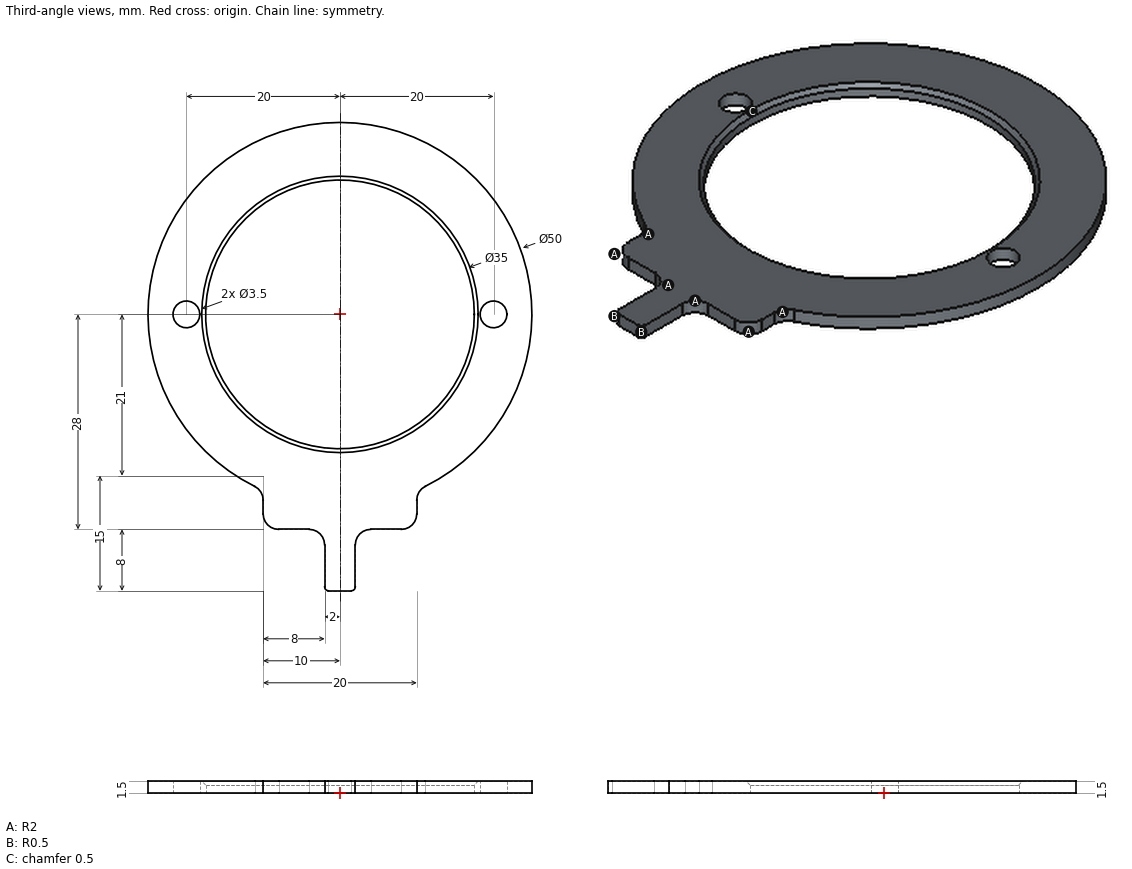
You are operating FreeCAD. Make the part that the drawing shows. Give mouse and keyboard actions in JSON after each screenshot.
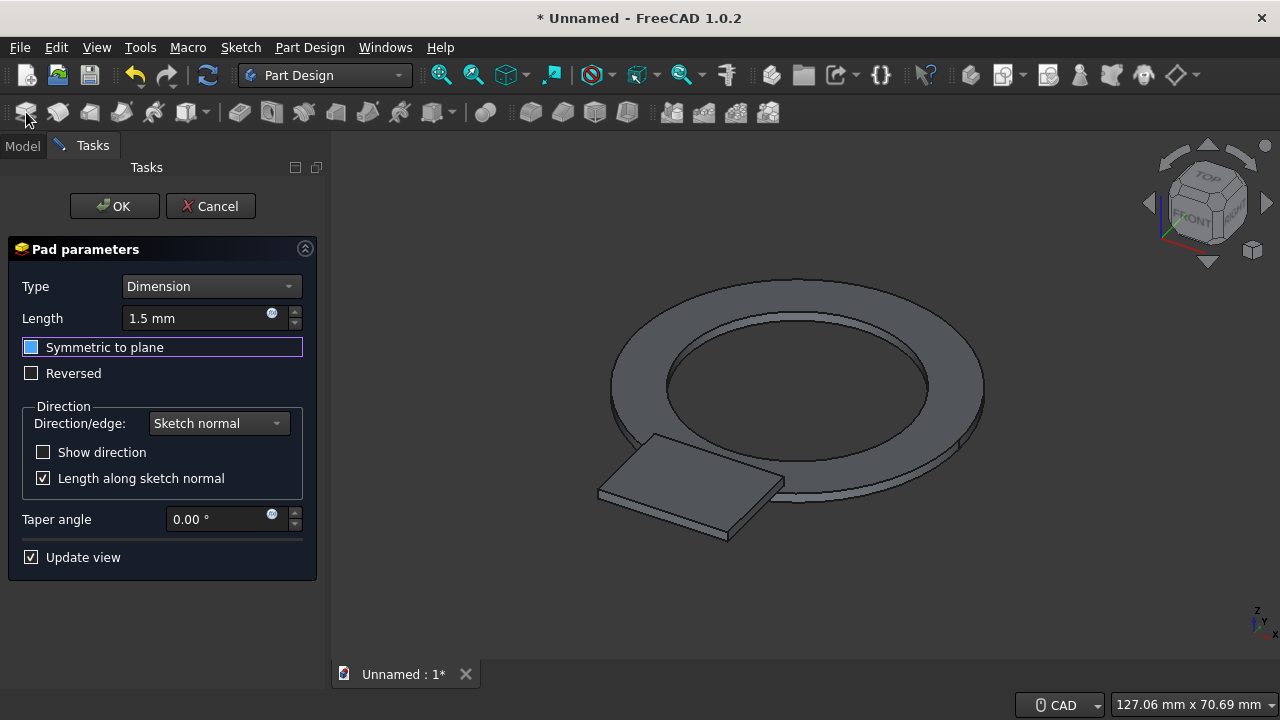
{"action": "left_click", "coordinate": [30, 373]}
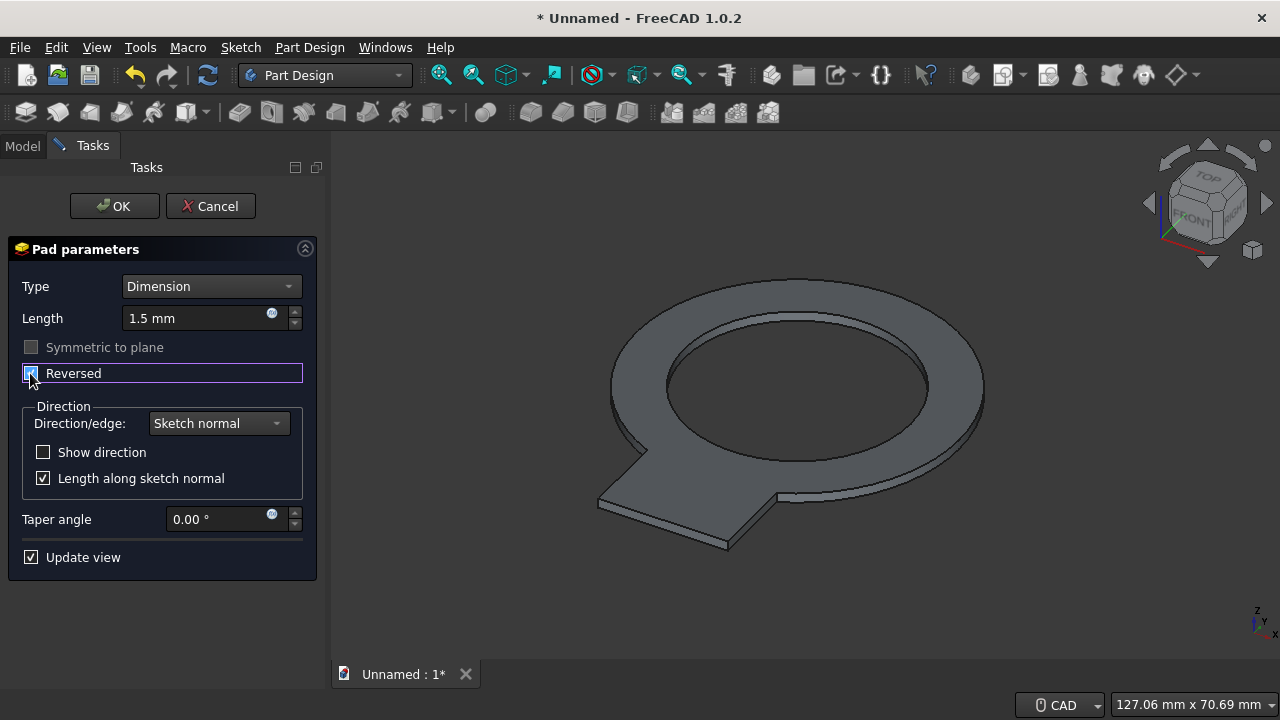
{"action": "left_click", "coordinate": [115, 206]}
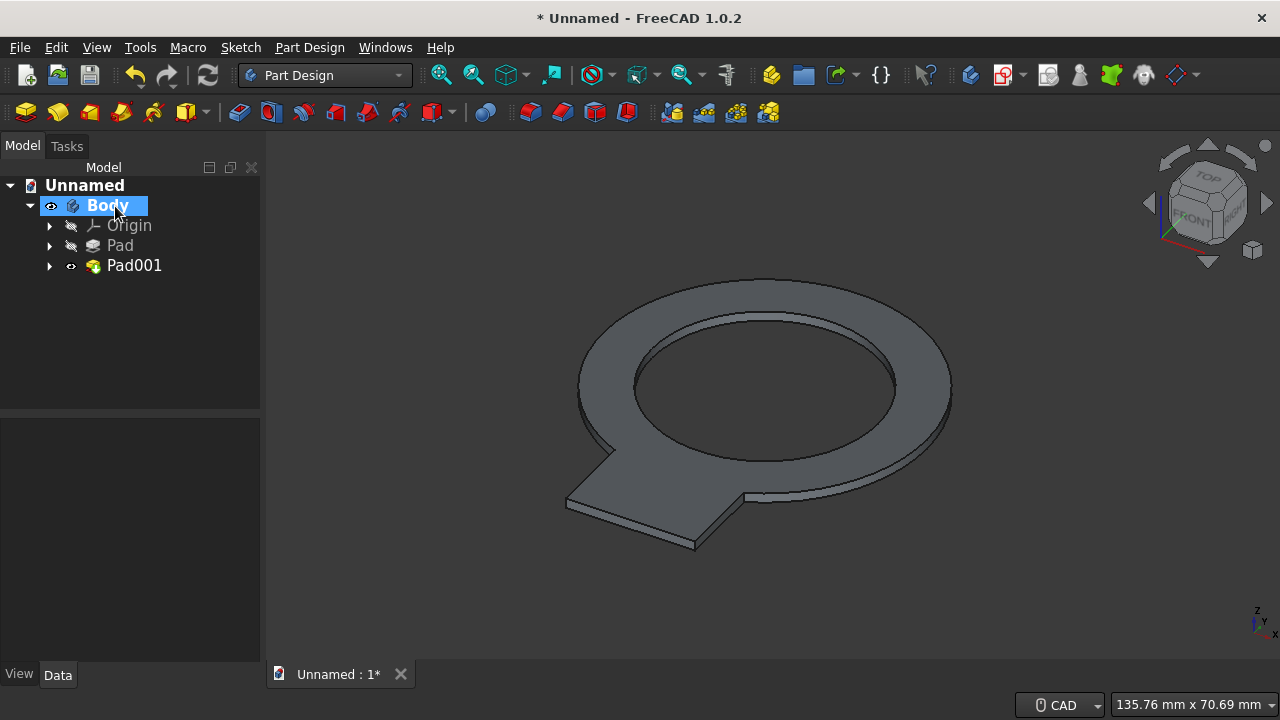
{"action": "left_click", "coordinate": [679, 471]}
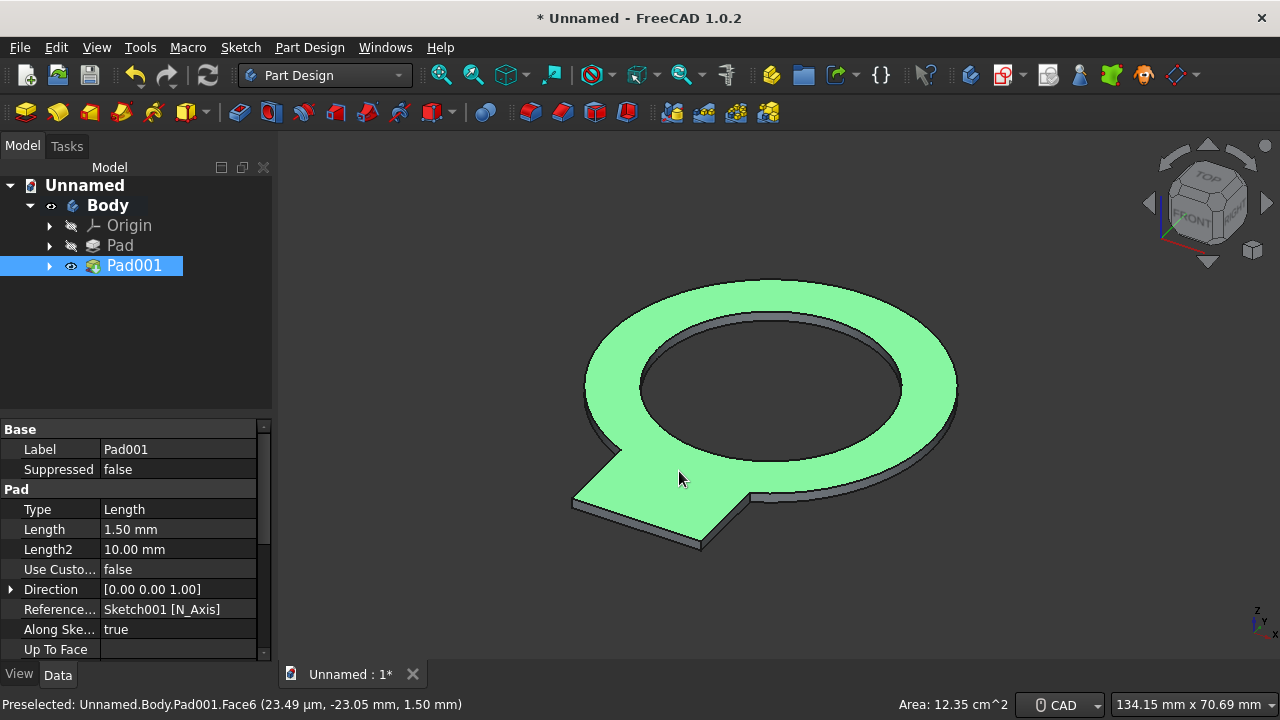
{"action": "left_click", "coordinate": [1004, 76]}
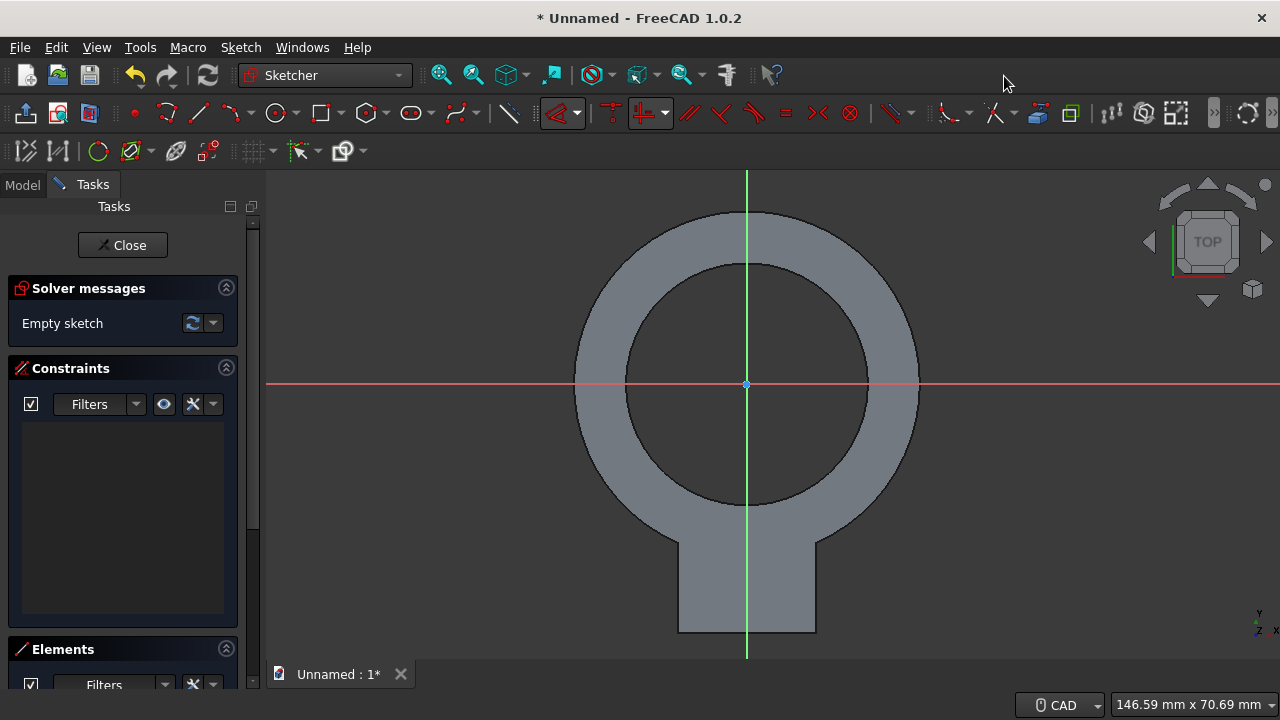
{"action": "scroll", "coordinate": [513, 198], "scroll_direction": "down", "scroll_amount": 1}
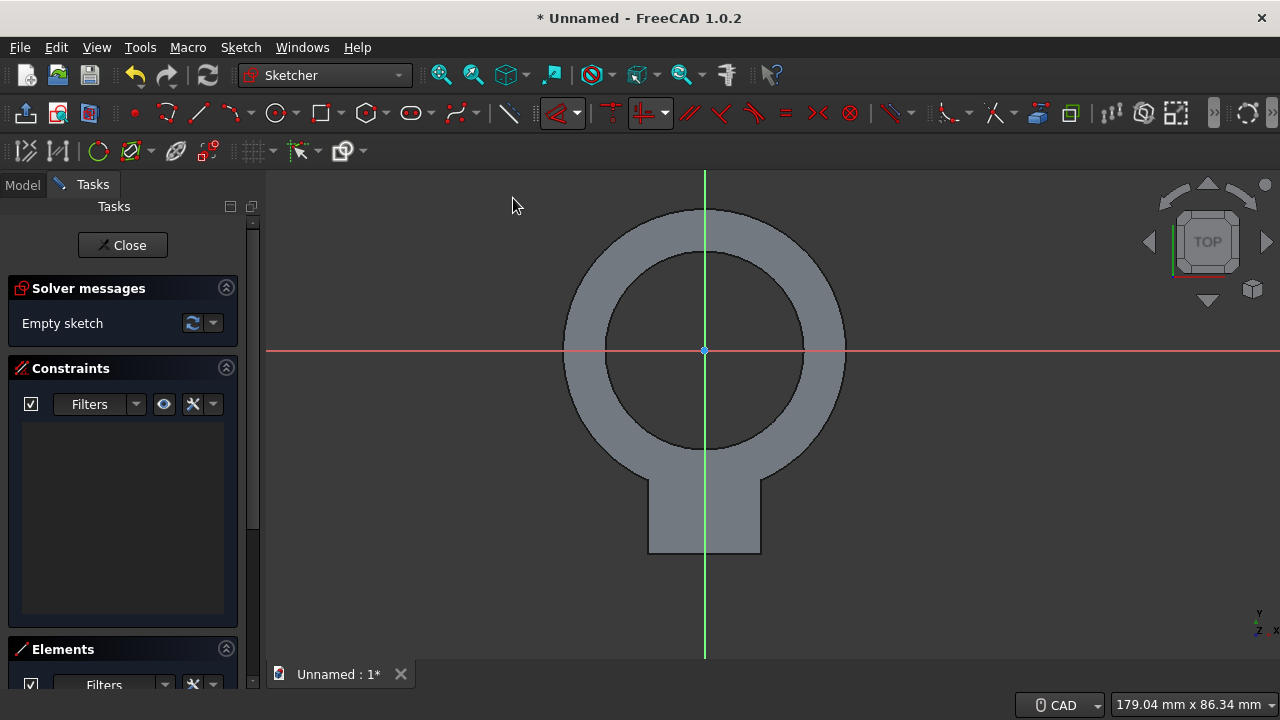
{"action": "scroll", "coordinate": [705, 530], "scroll_direction": "up", "scroll_amount": 2}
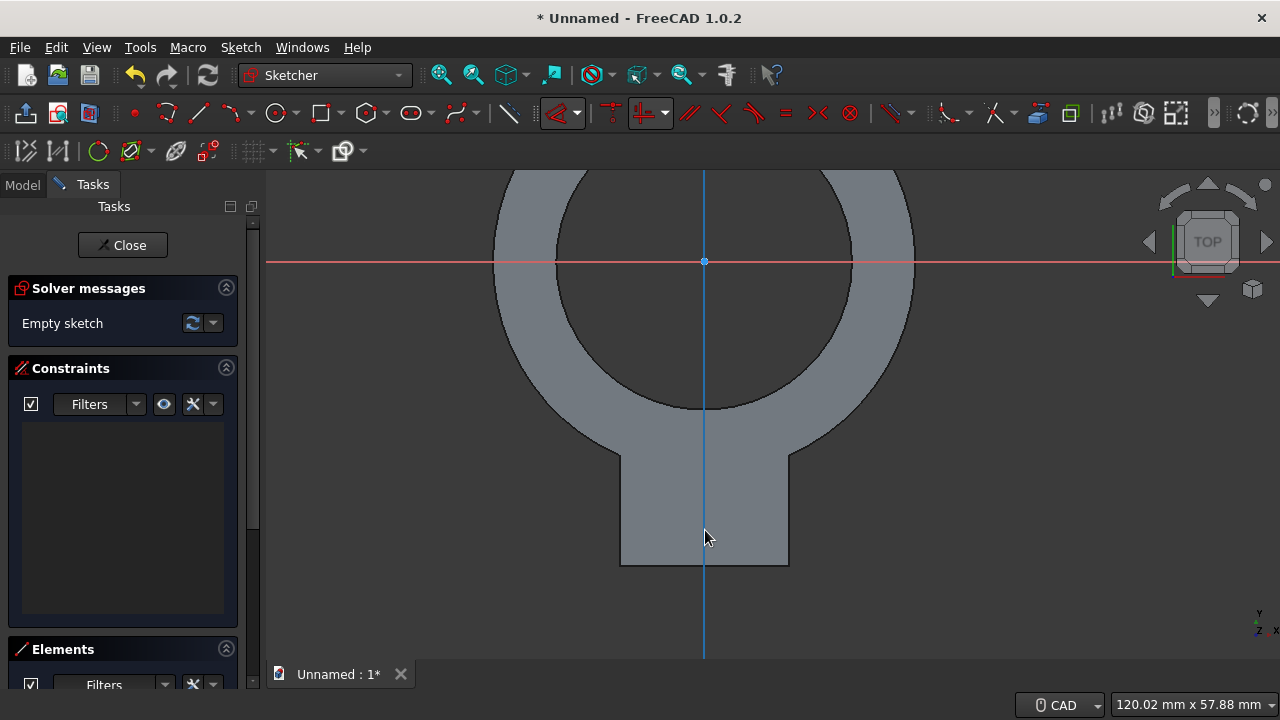
{"action": "left_click", "coordinate": [322, 114]}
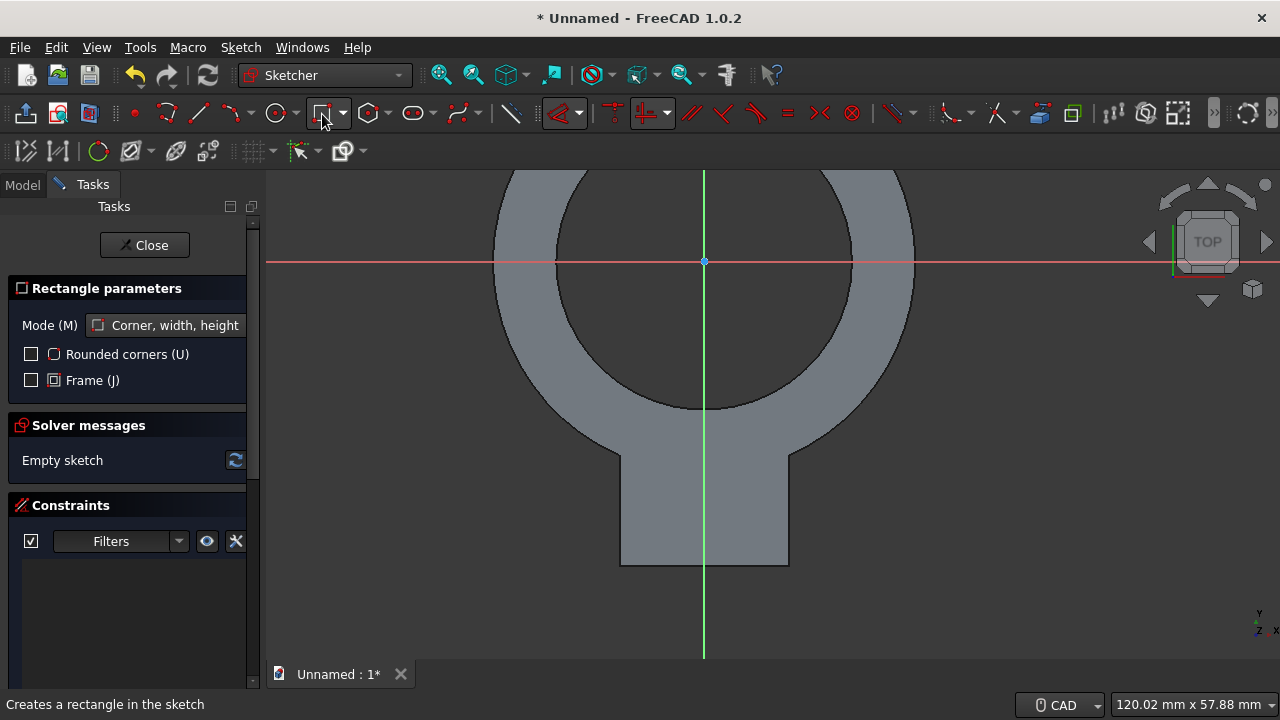
{"action": "left_click", "coordinate": [620, 498]}
{"action": "left_click", "coordinate": [687, 566]}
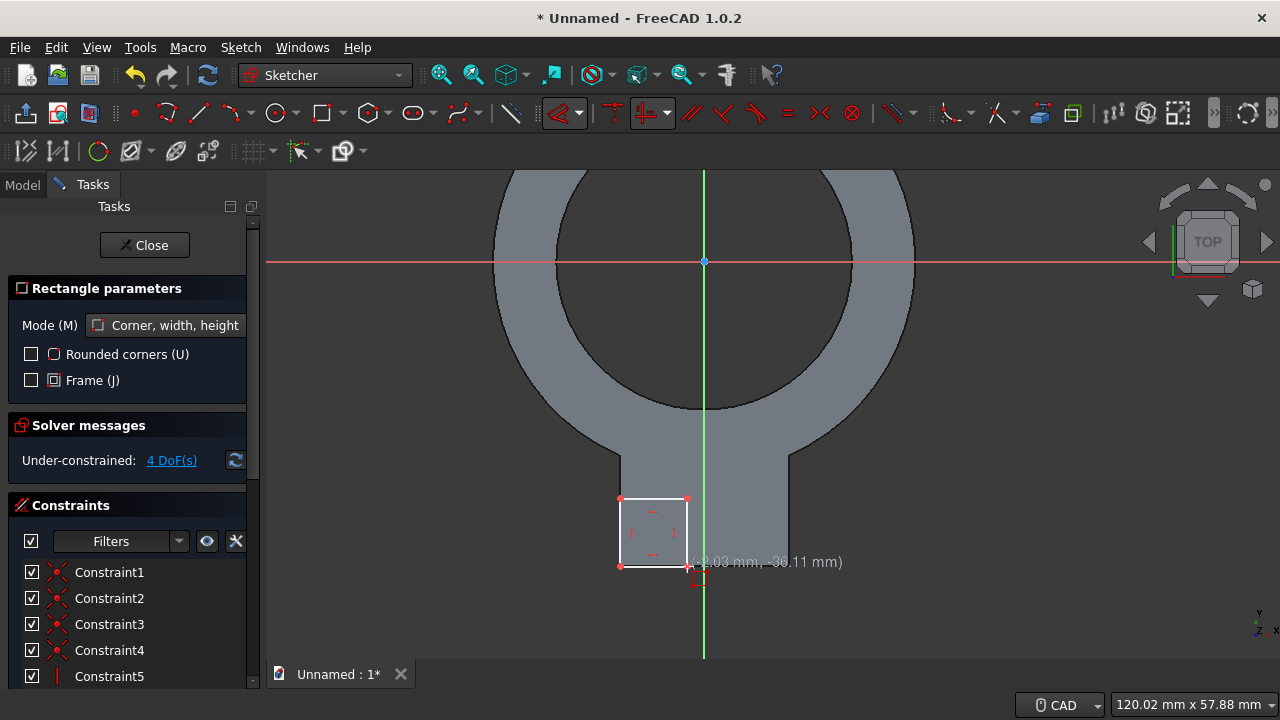
{"action": "left_click", "coordinate": [721, 498]}
{"action": "left_click", "coordinate": [789, 566]}
{"action": "key", "text": "Escape"}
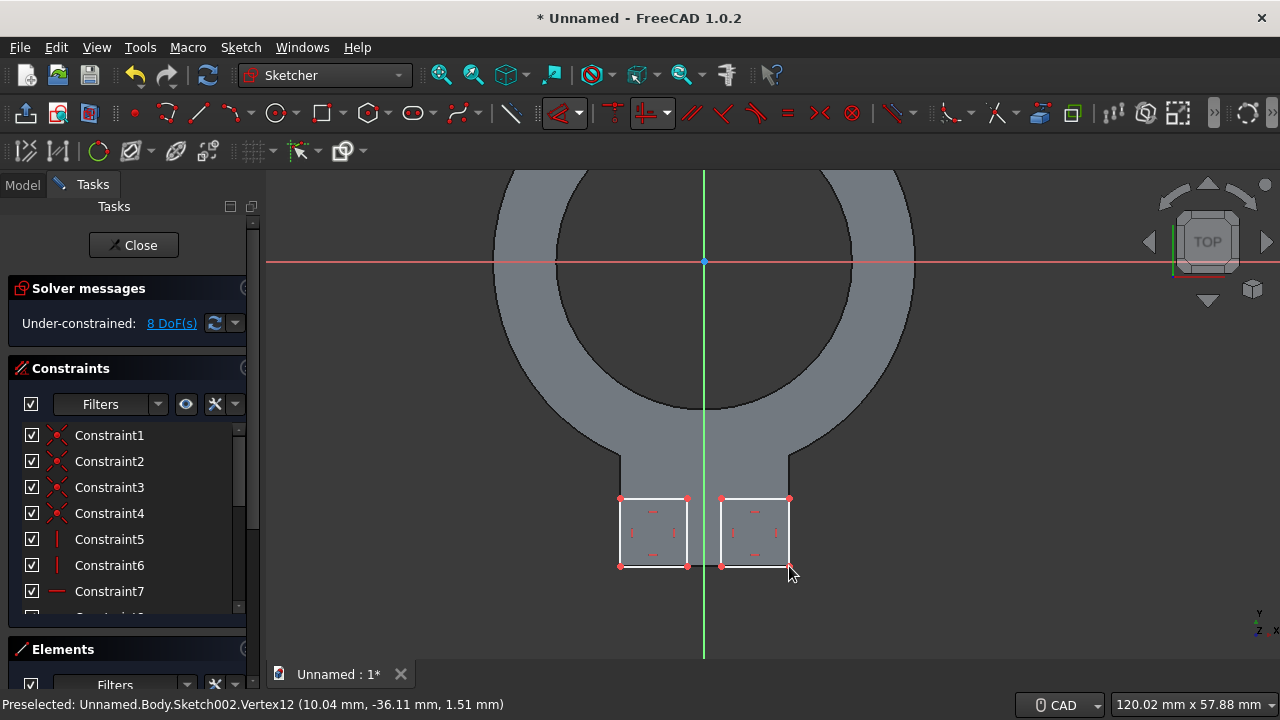
{"action": "left_click", "coordinate": [687, 499]}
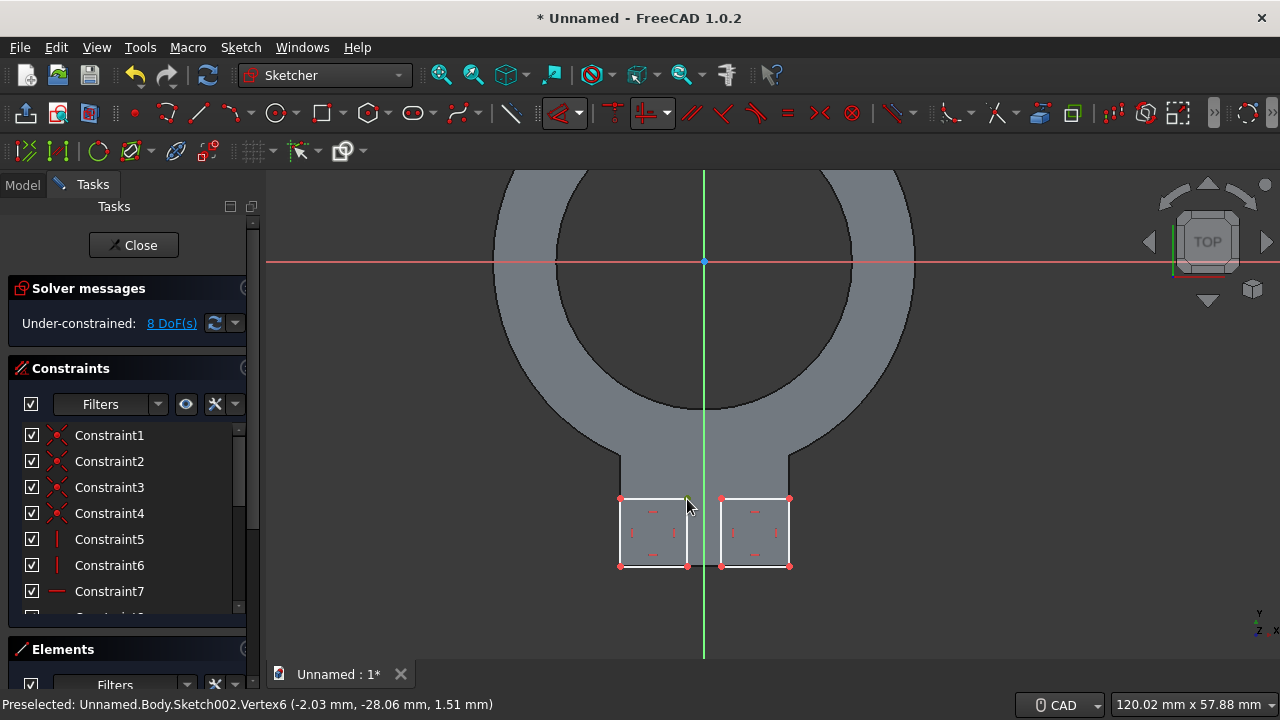
{"action": "left_click", "coordinate": [721, 499]}